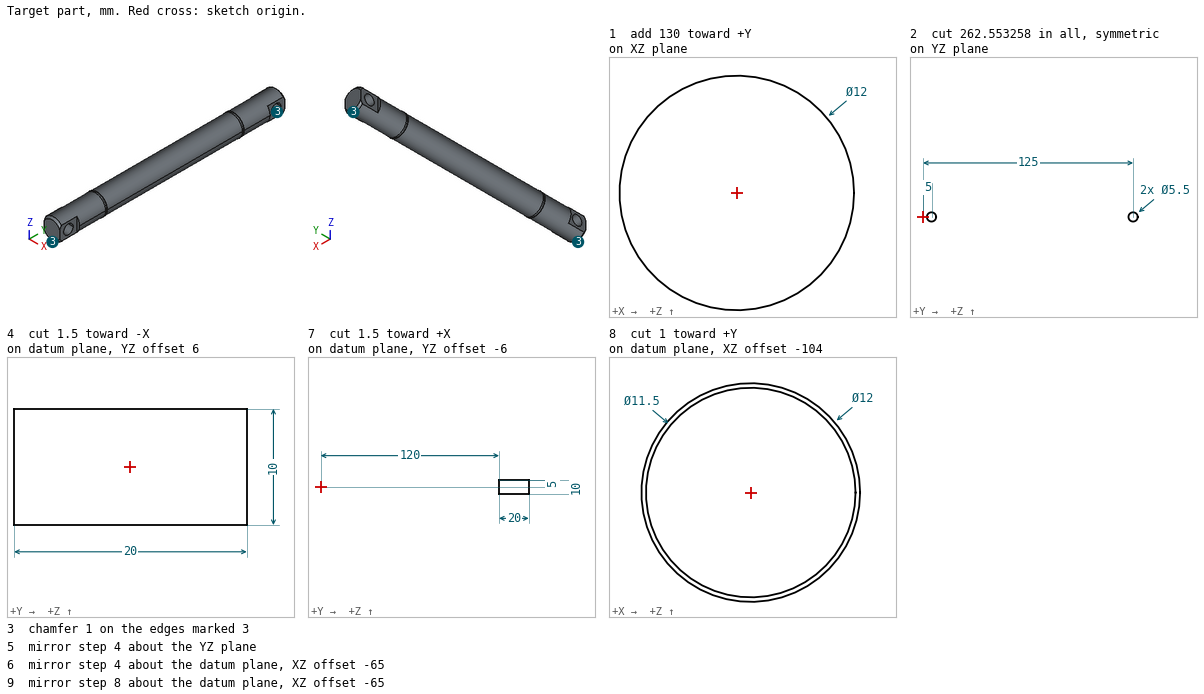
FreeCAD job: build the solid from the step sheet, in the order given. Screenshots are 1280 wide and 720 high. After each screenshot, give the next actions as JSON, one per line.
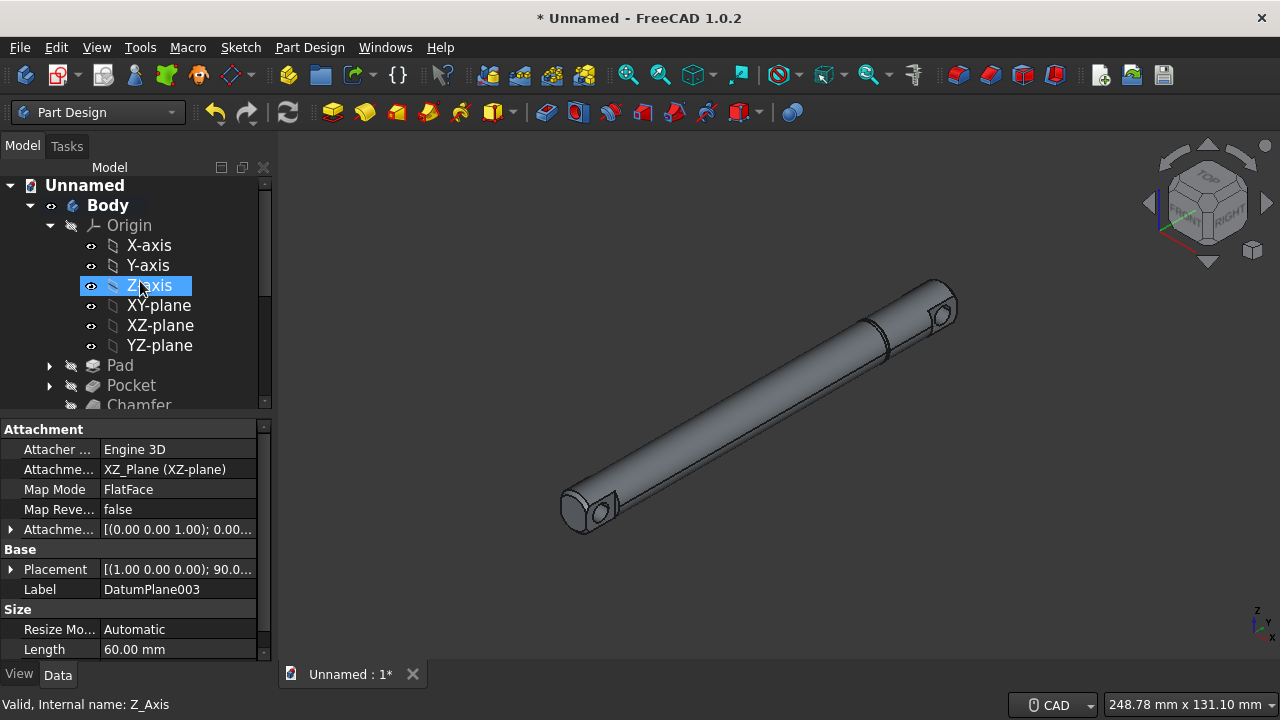
{"action": "left_click", "coordinate": [136, 326]}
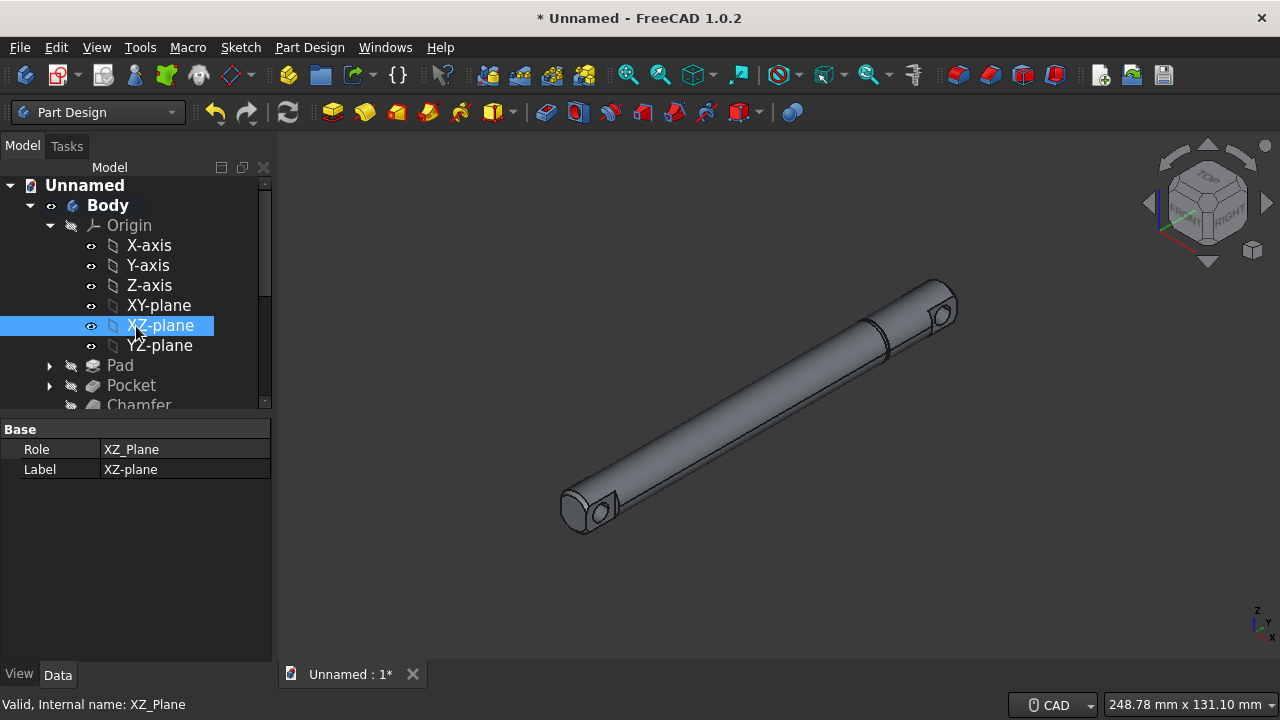
{"action": "left_click", "coordinate": [232, 76]}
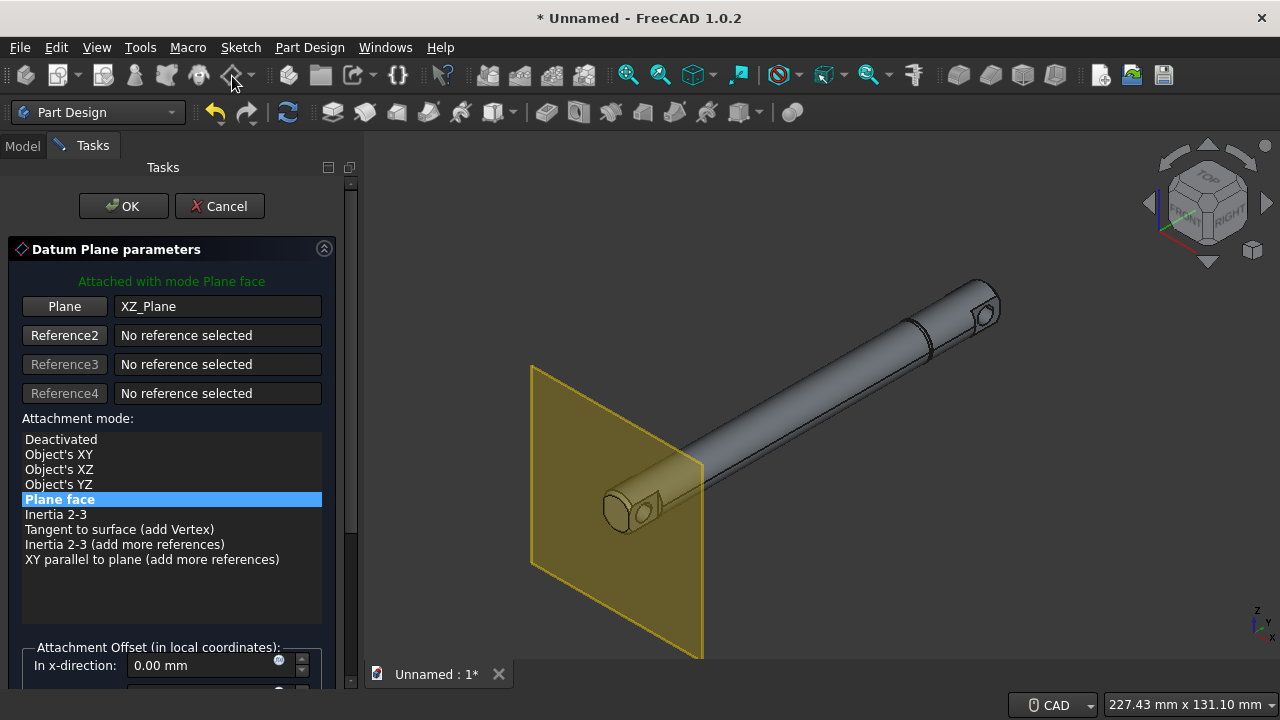
{"action": "scroll", "coordinate": [351, 432], "scroll_direction": "down", "scroll_amount": 2}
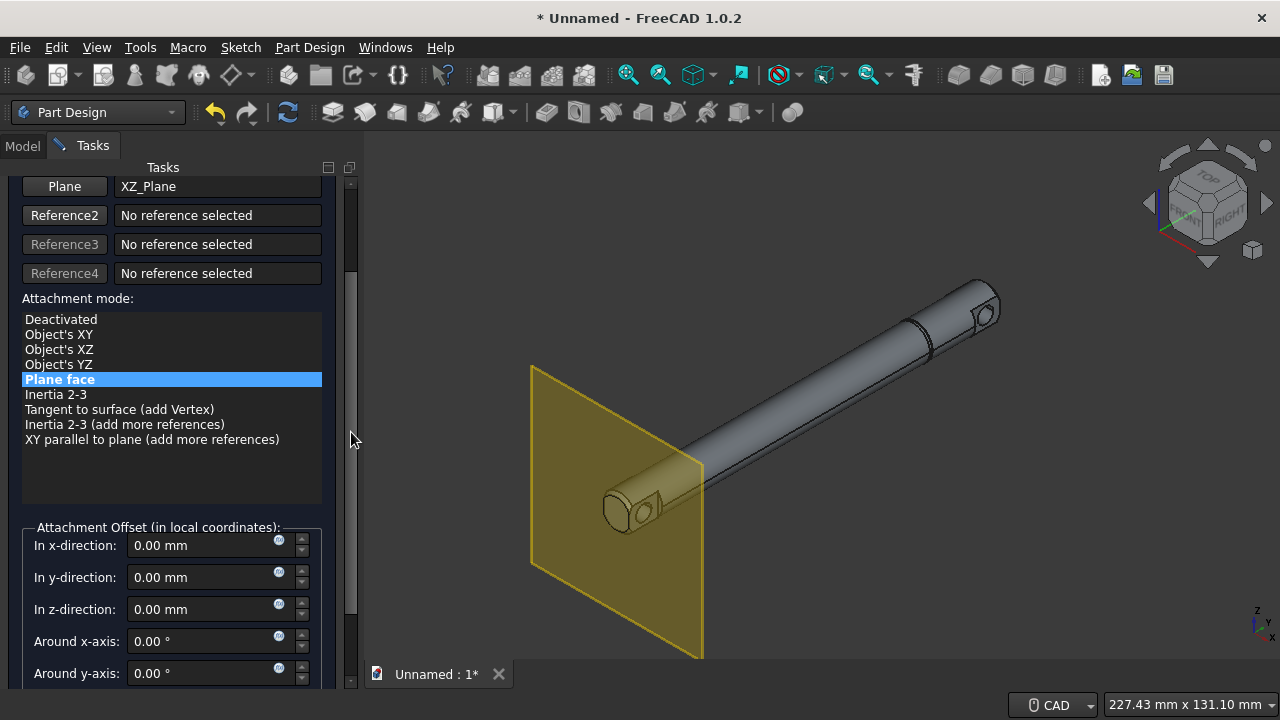
{"action": "triple_click", "coordinate": [210, 609]}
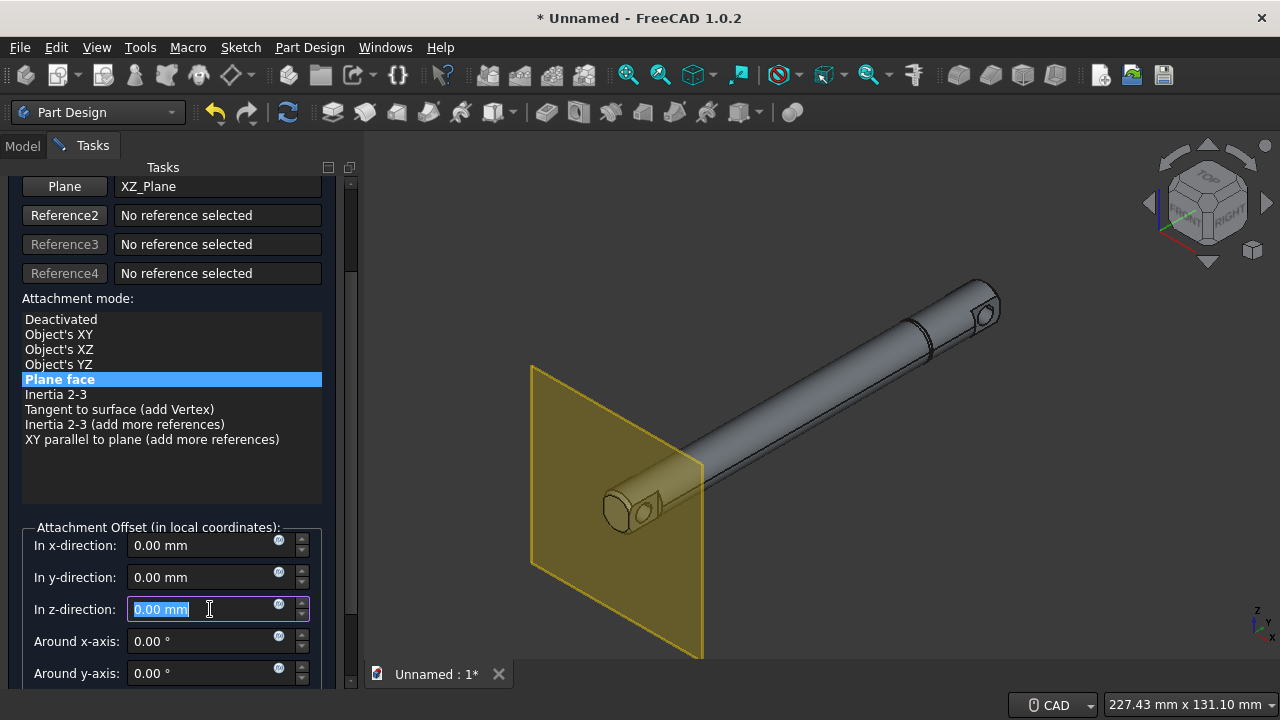
{"action": "type", "text": "-65"}
{"action": "key", "text": "Tab"}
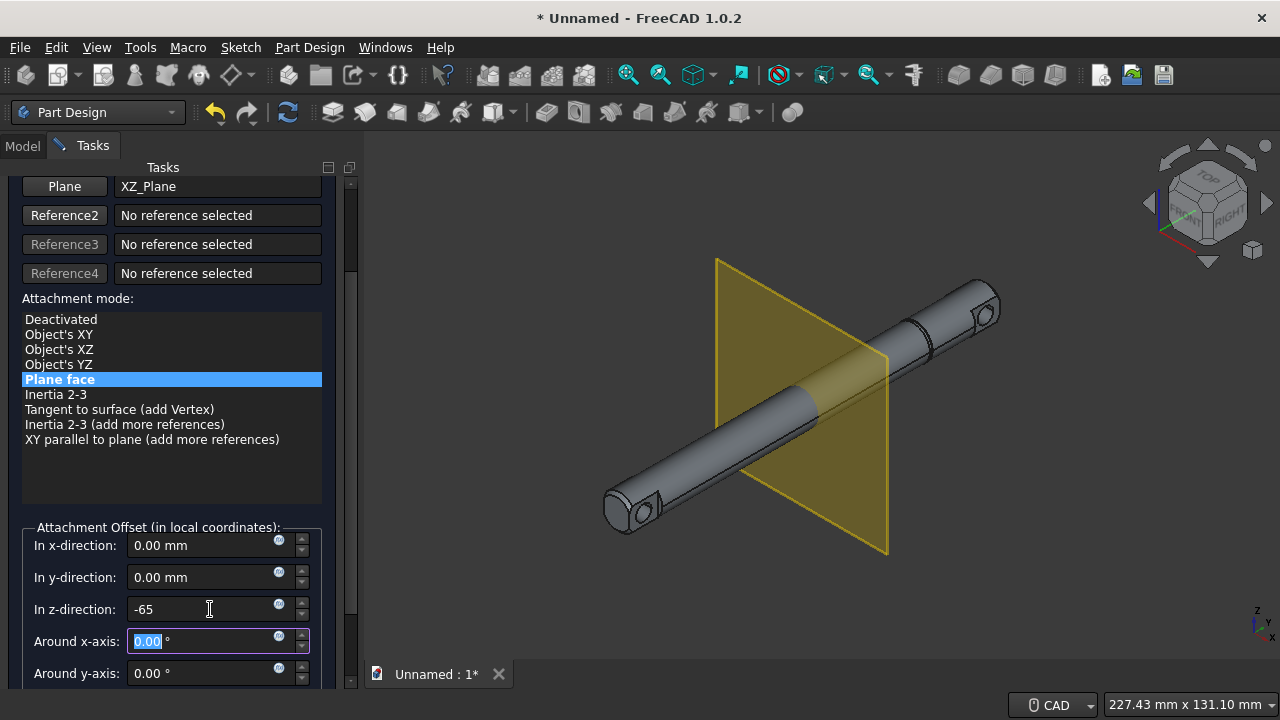
{"action": "scroll", "coordinate": [351, 432], "scroll_direction": "up", "scroll_amount": 3}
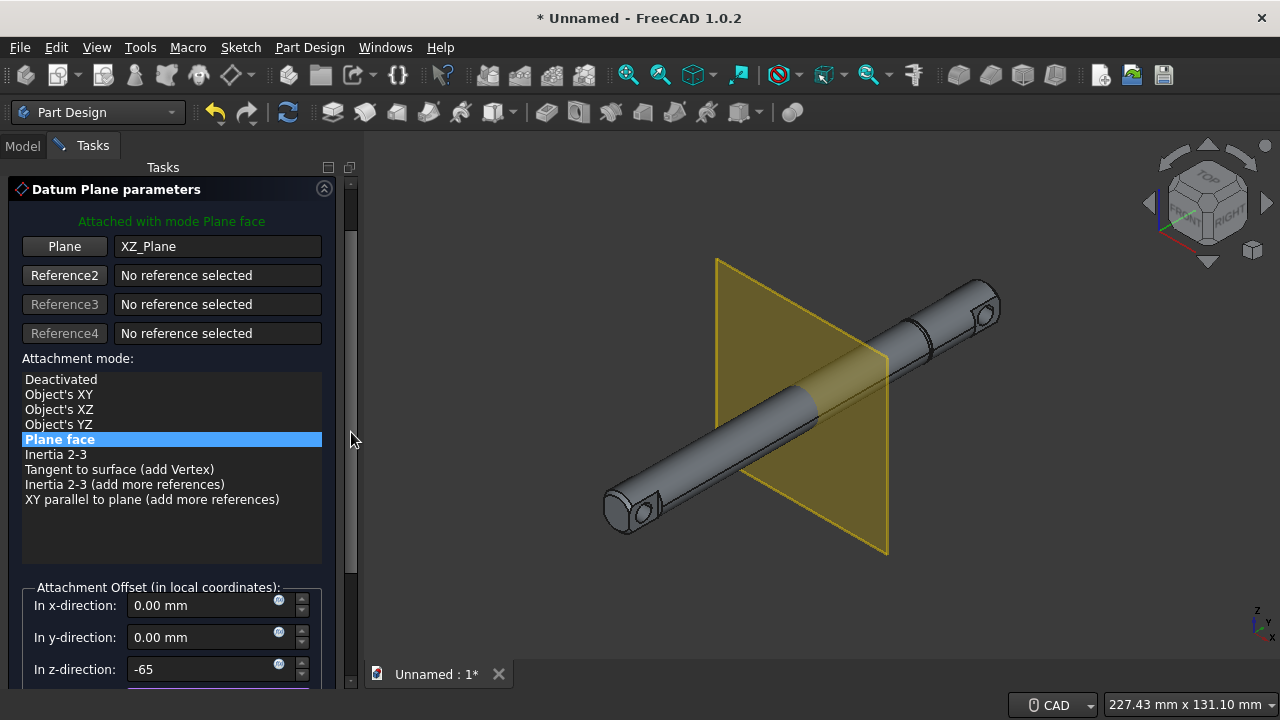
{"action": "left_click", "coordinate": [124, 206]}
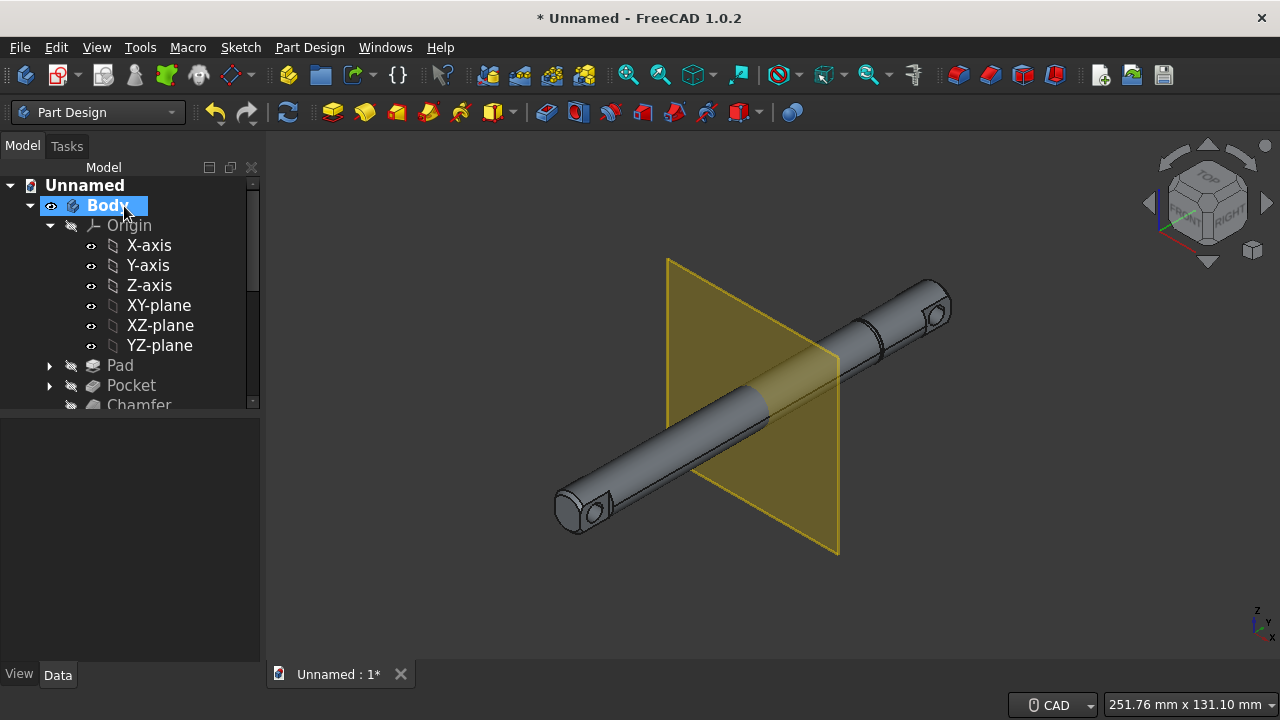
{"action": "scroll", "coordinate": [100, 301], "scroll_direction": "down", "scroll_amount": 3}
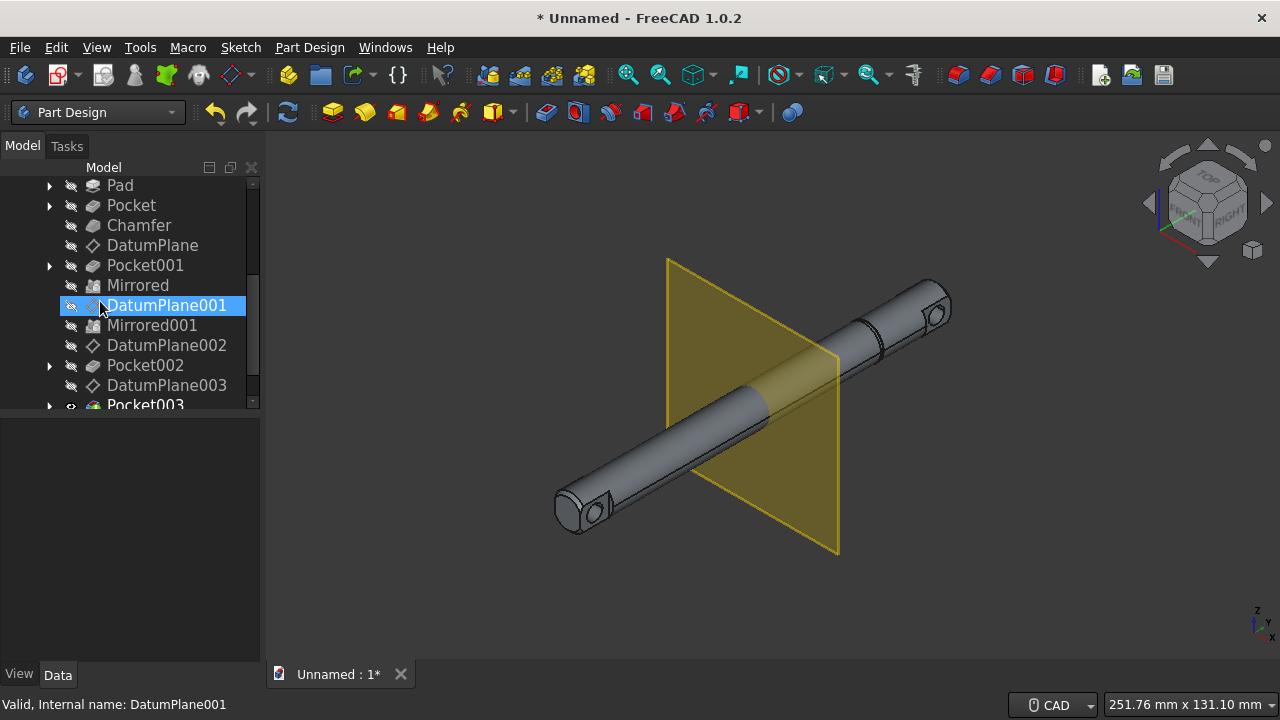
{"action": "left_click", "coordinate": [116, 406]}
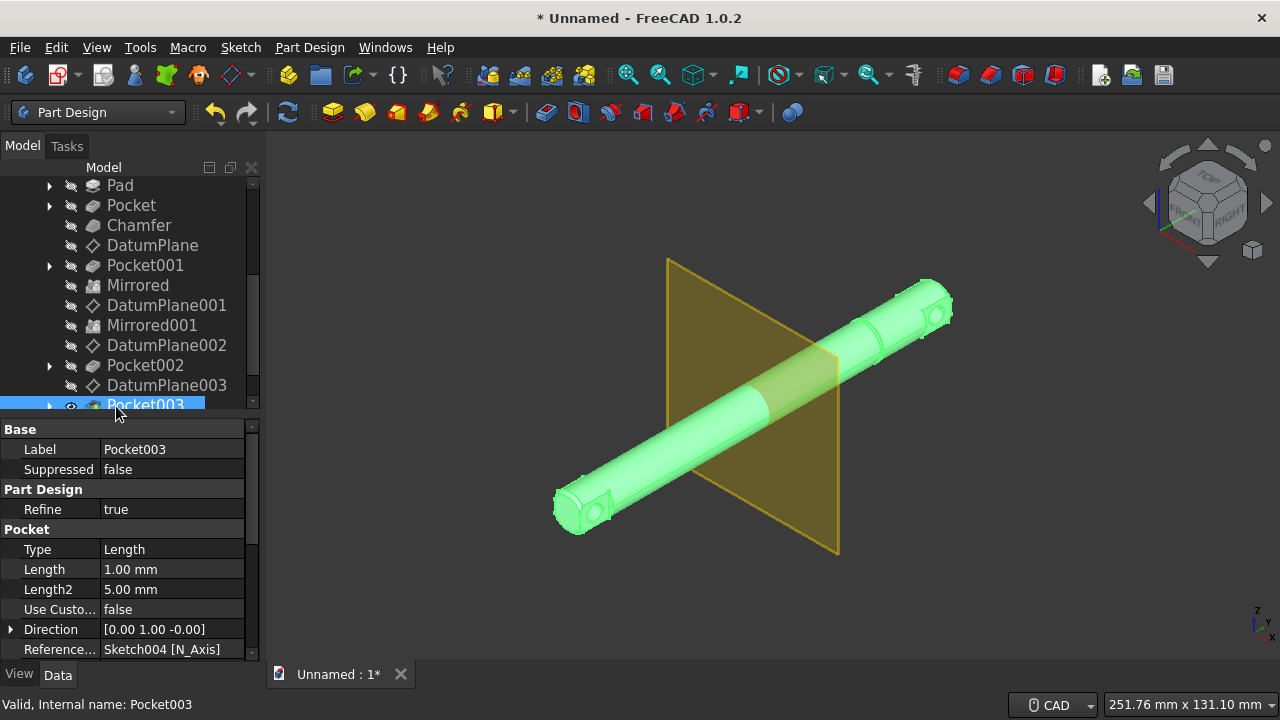
{"action": "left_click", "coordinate": [488, 76]}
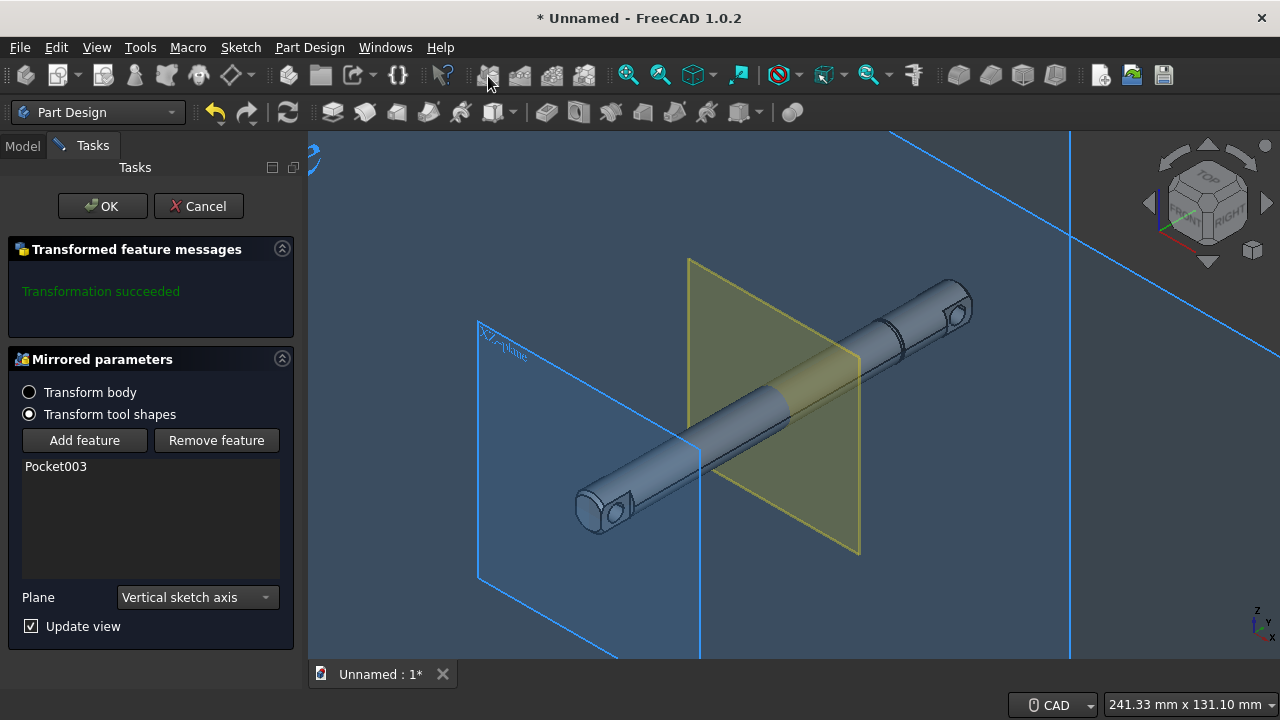
{"action": "left_click", "coordinate": [198, 598]}